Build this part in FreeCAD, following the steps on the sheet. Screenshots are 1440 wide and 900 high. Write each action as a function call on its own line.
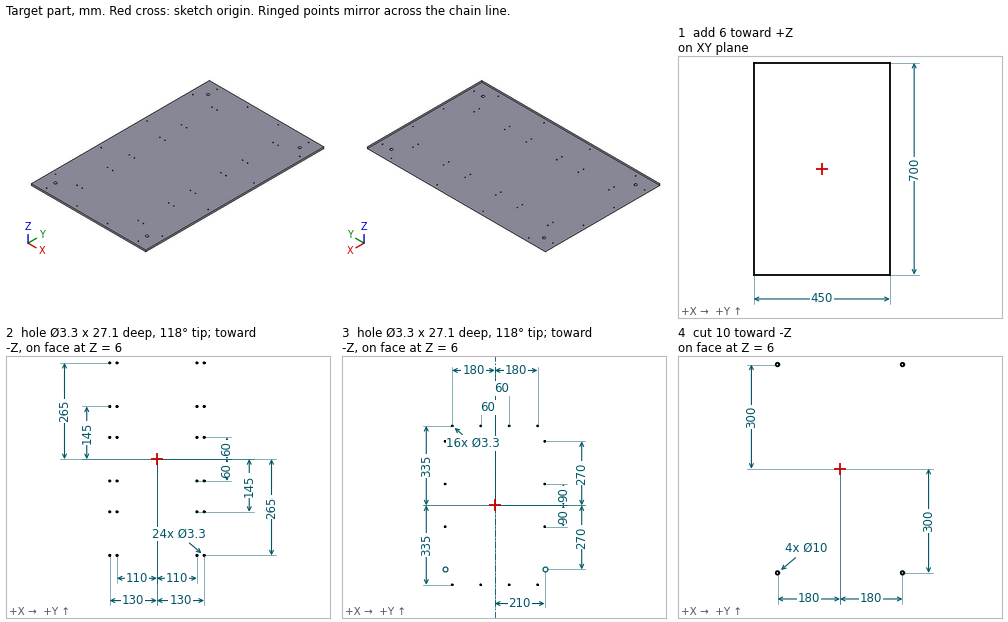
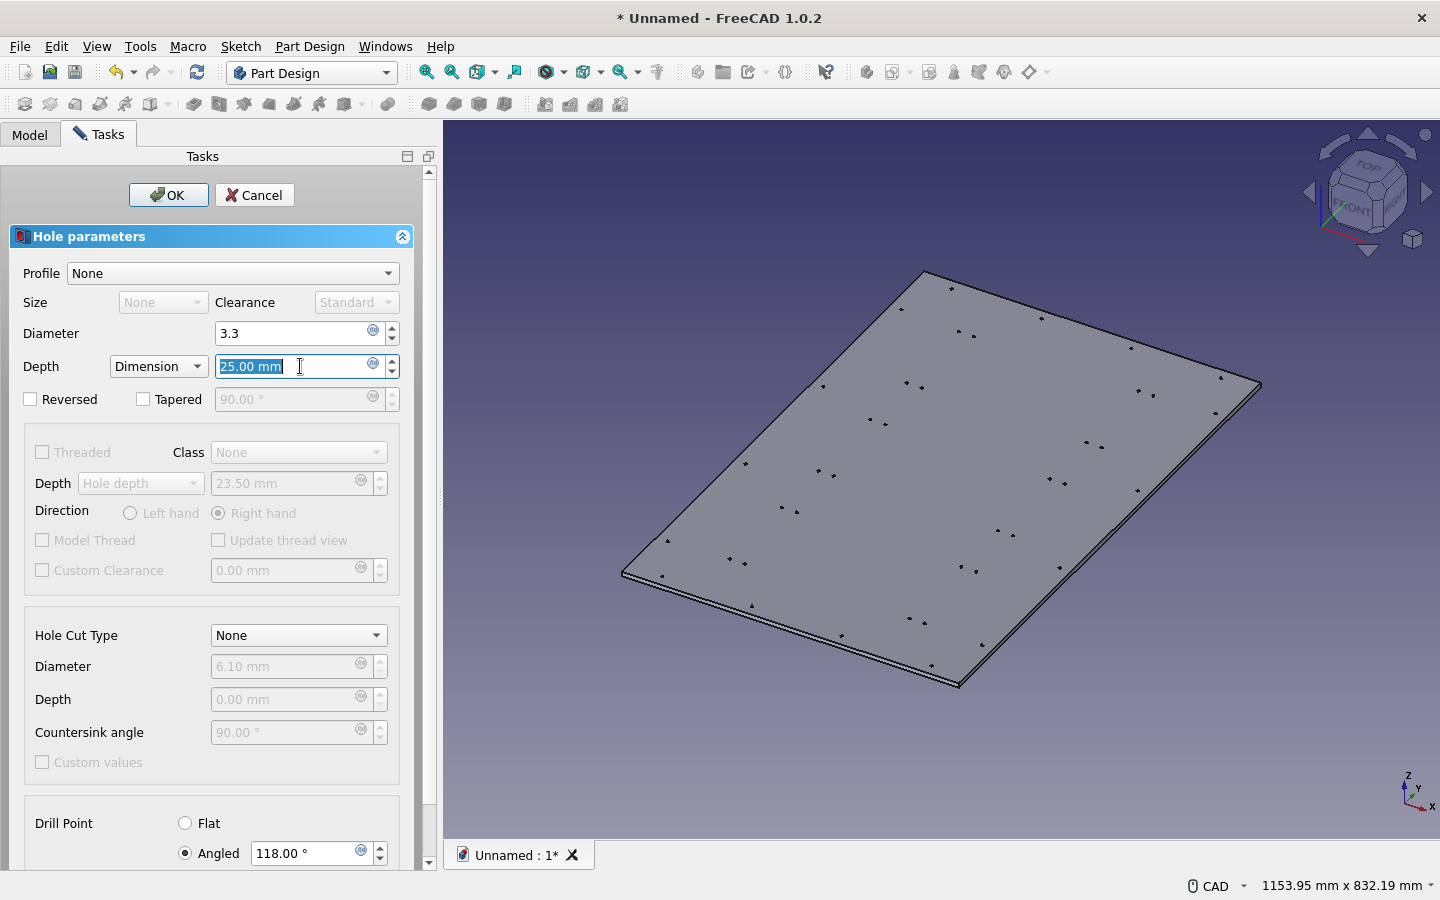
text(27.1)
key(Tab)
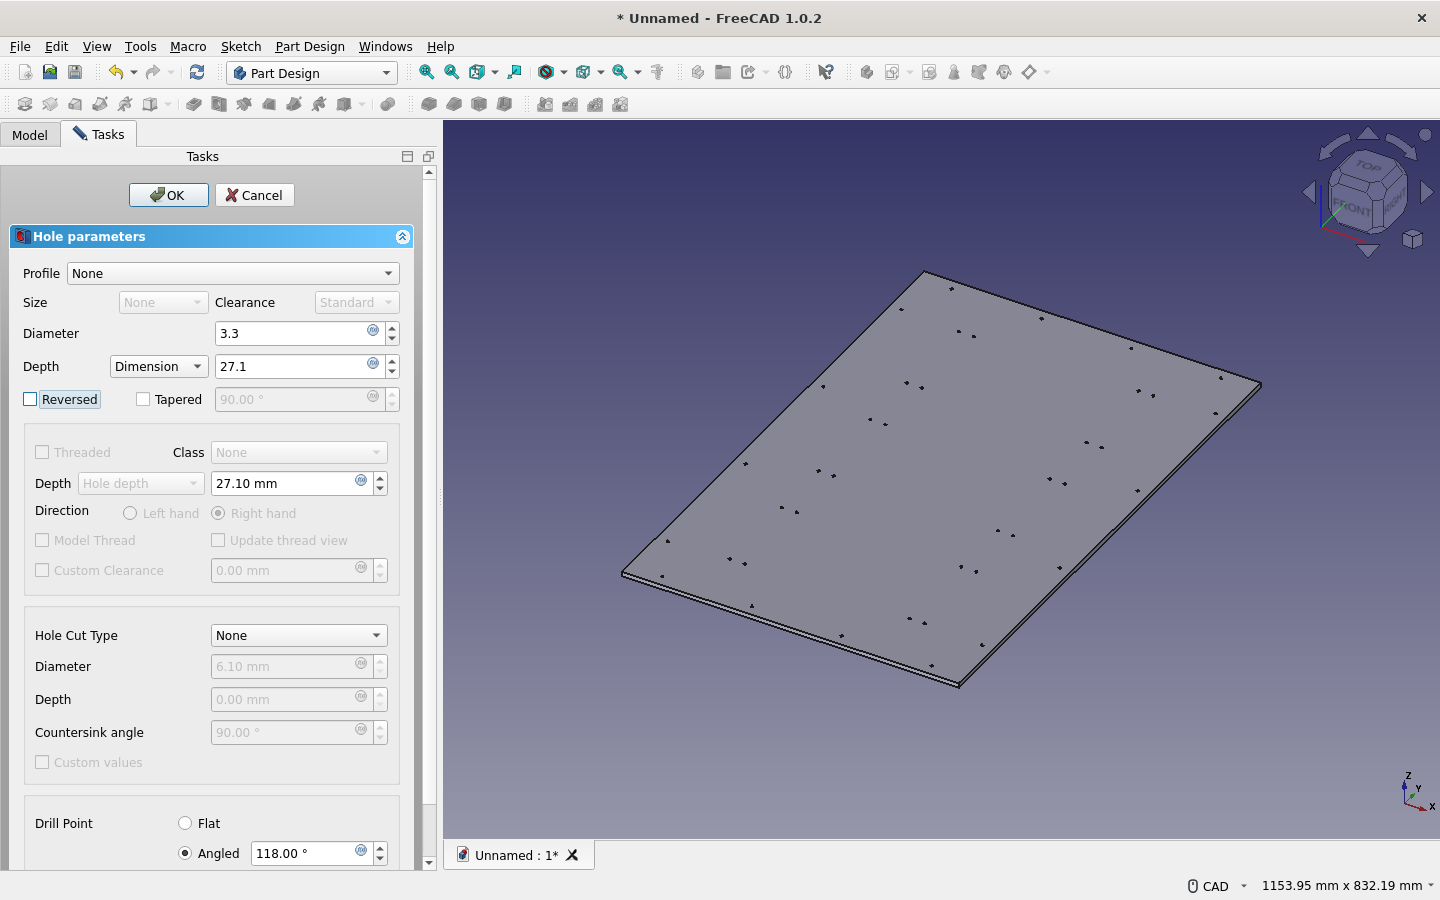
click(169, 195)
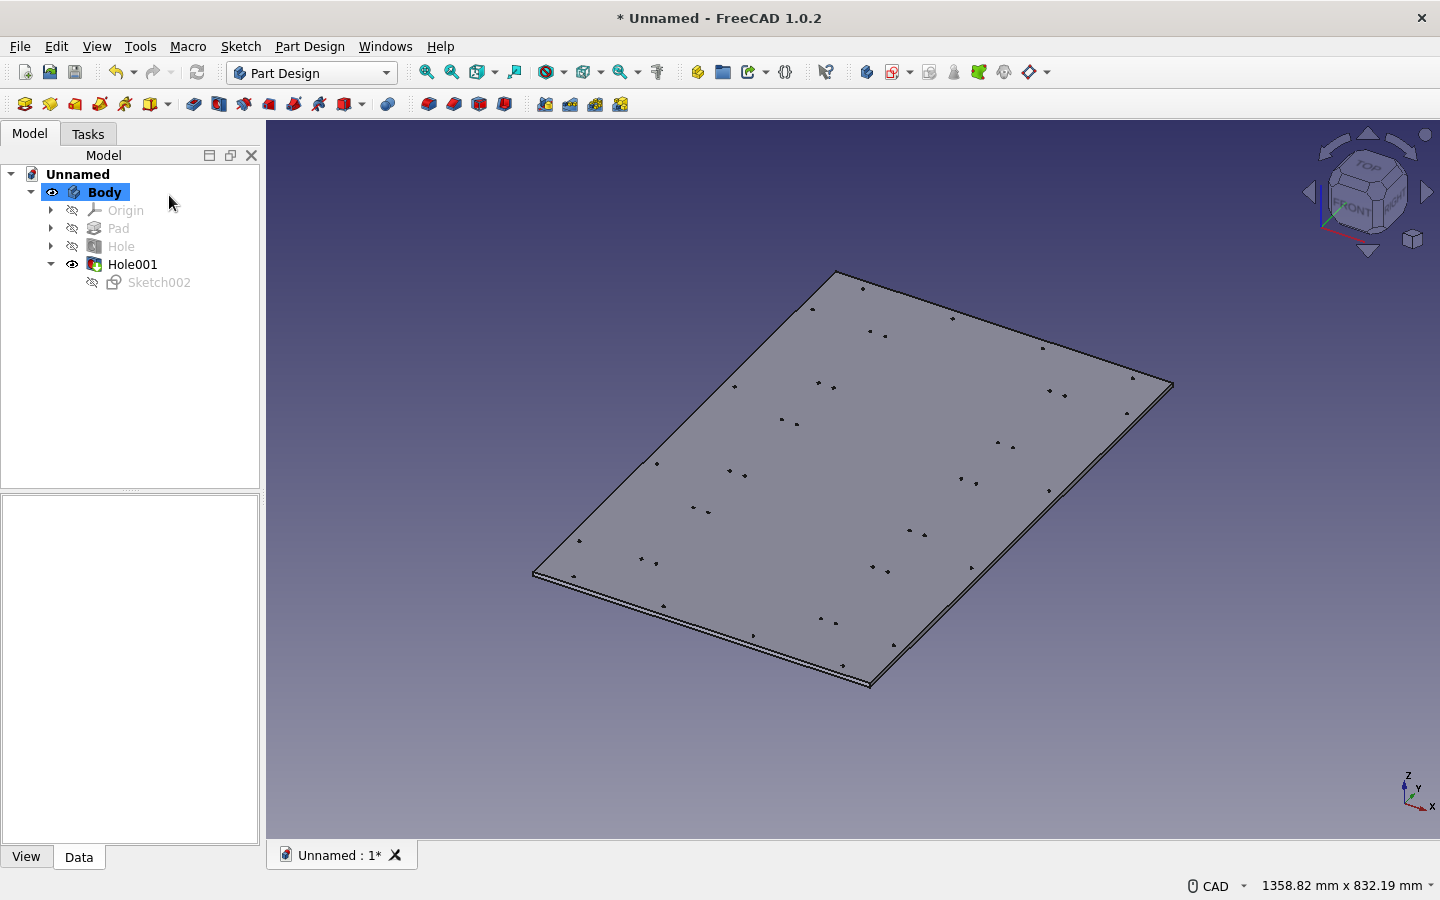
click(853, 476)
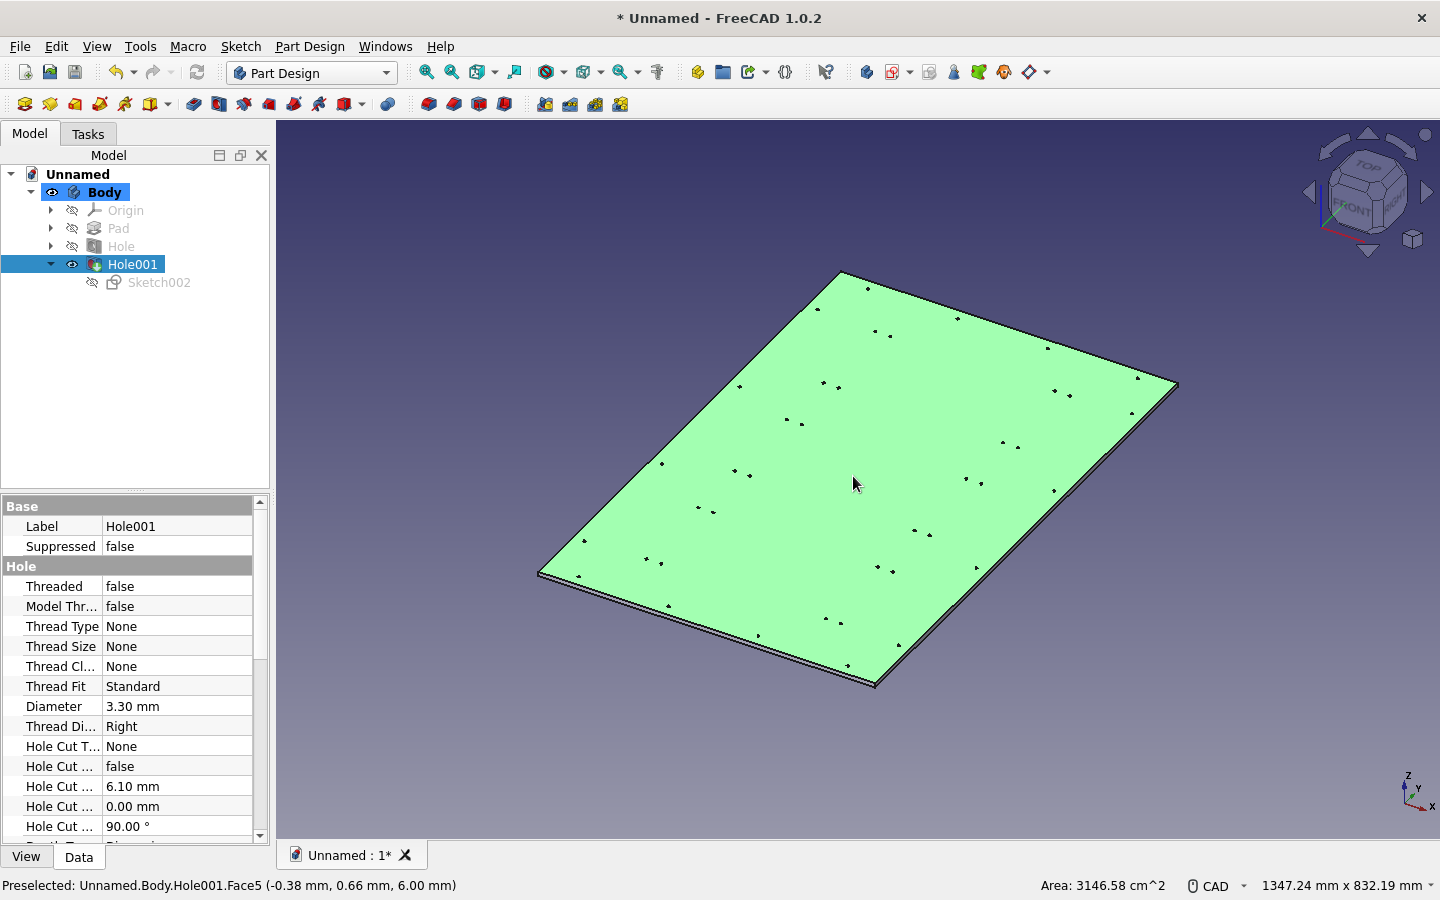
click(892, 72)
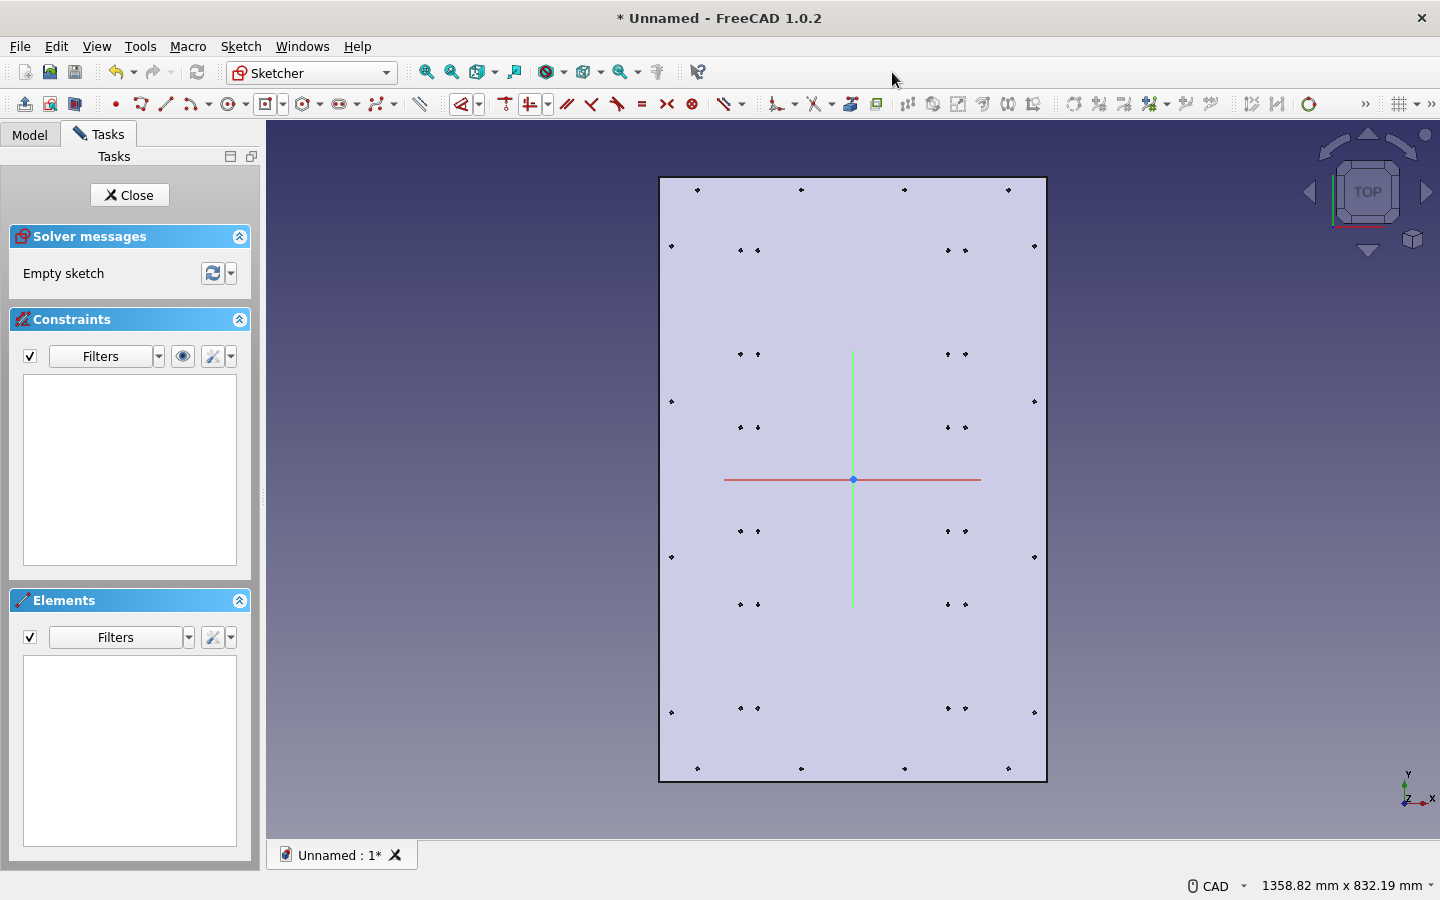
click(228, 104)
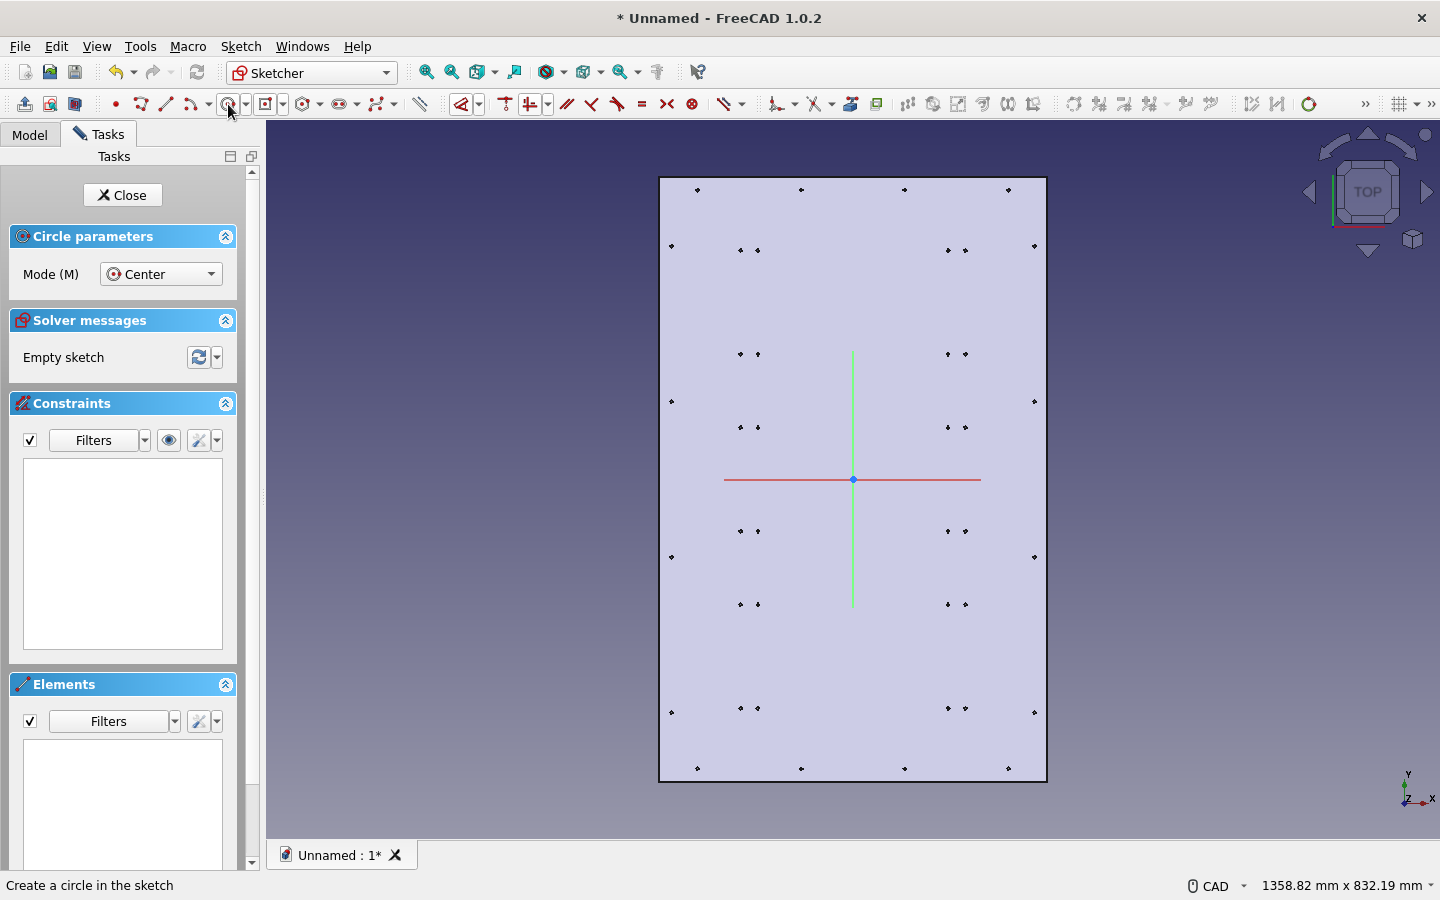
scroll(1009, 739, up, 9)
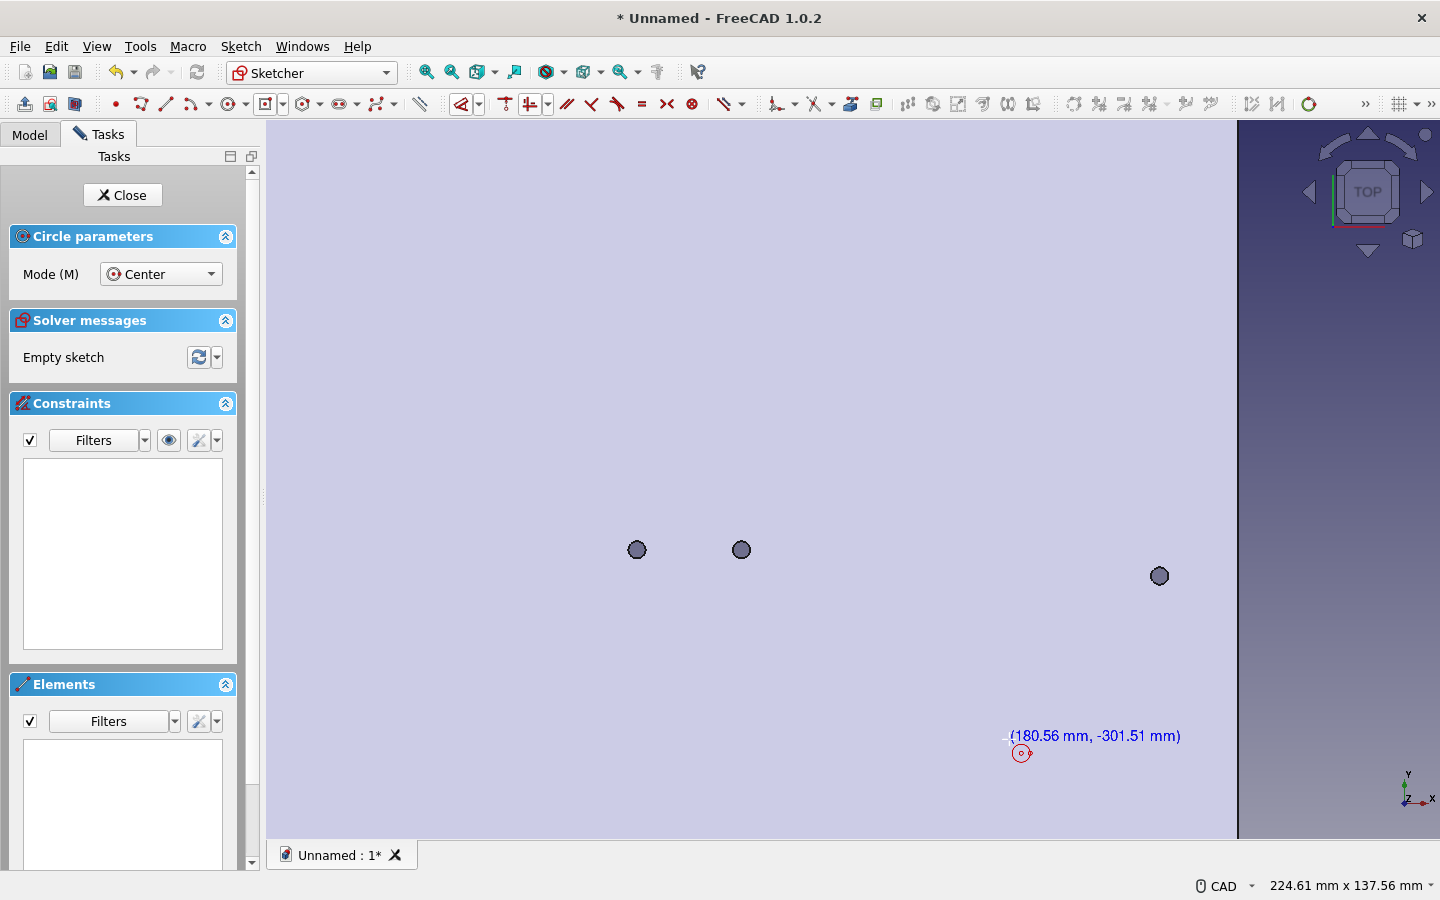
scroll(898, 685, down, 10)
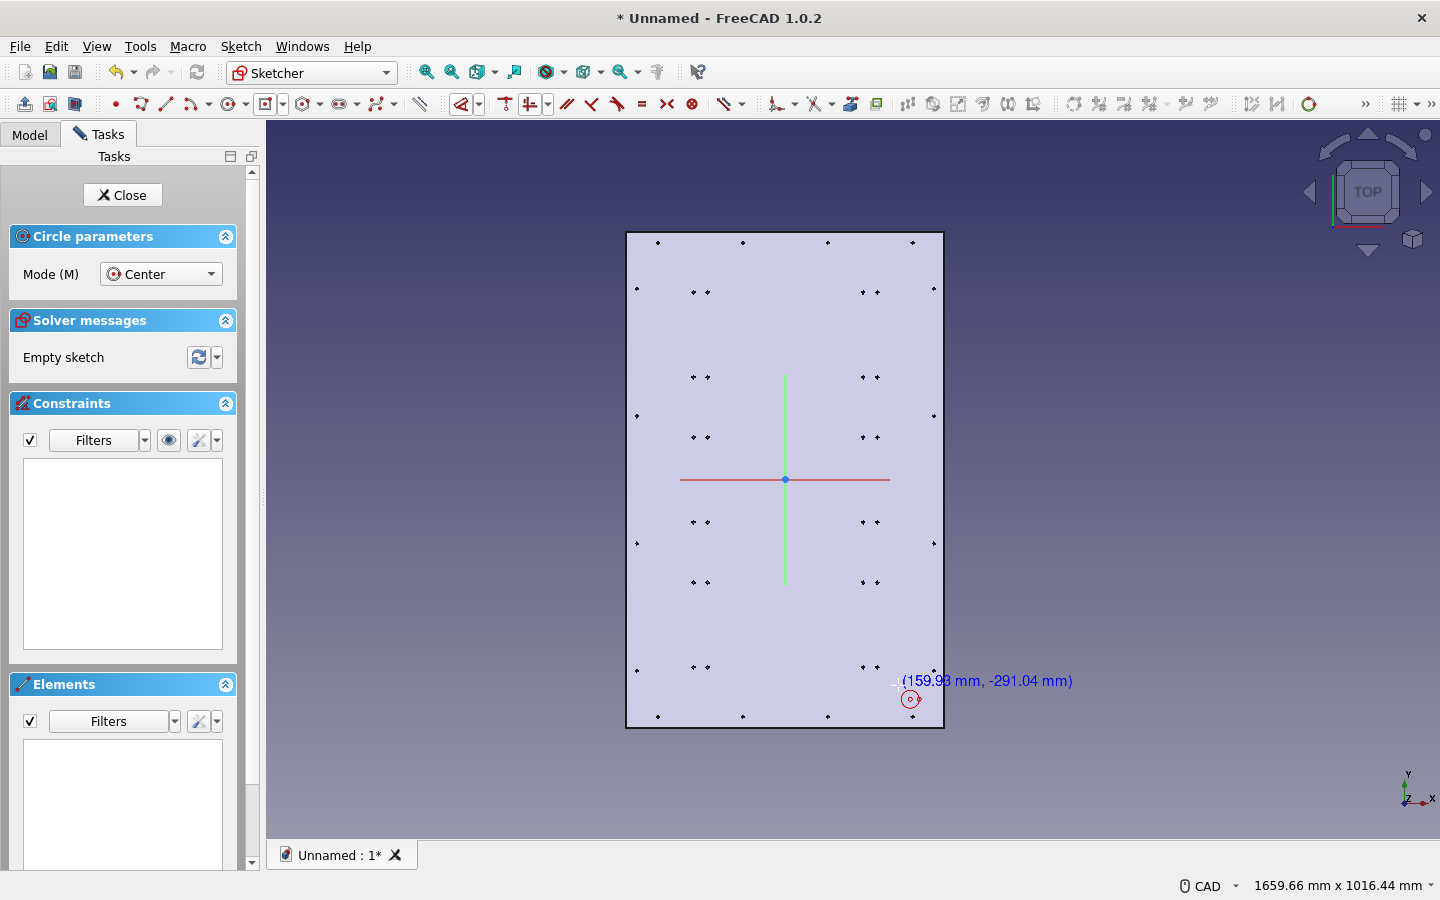
click(913, 692)
move(915, 690)